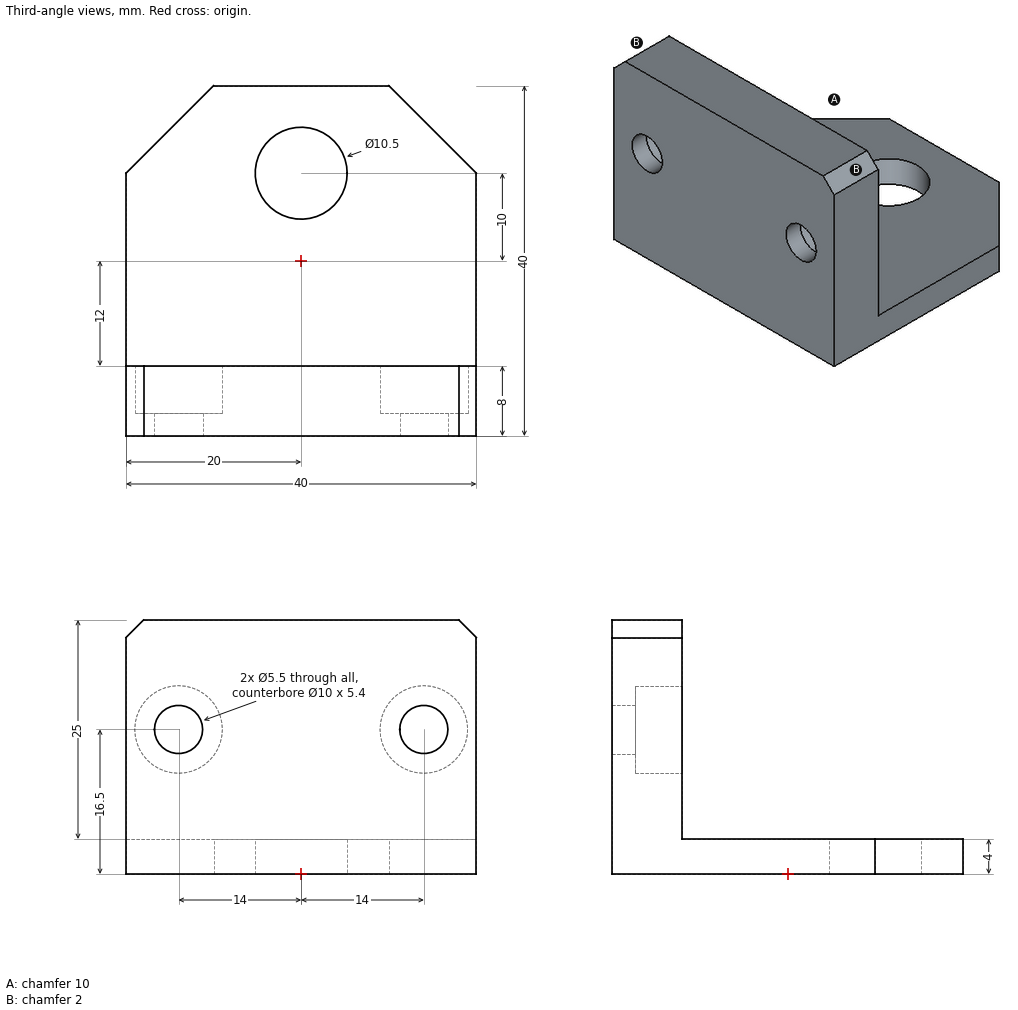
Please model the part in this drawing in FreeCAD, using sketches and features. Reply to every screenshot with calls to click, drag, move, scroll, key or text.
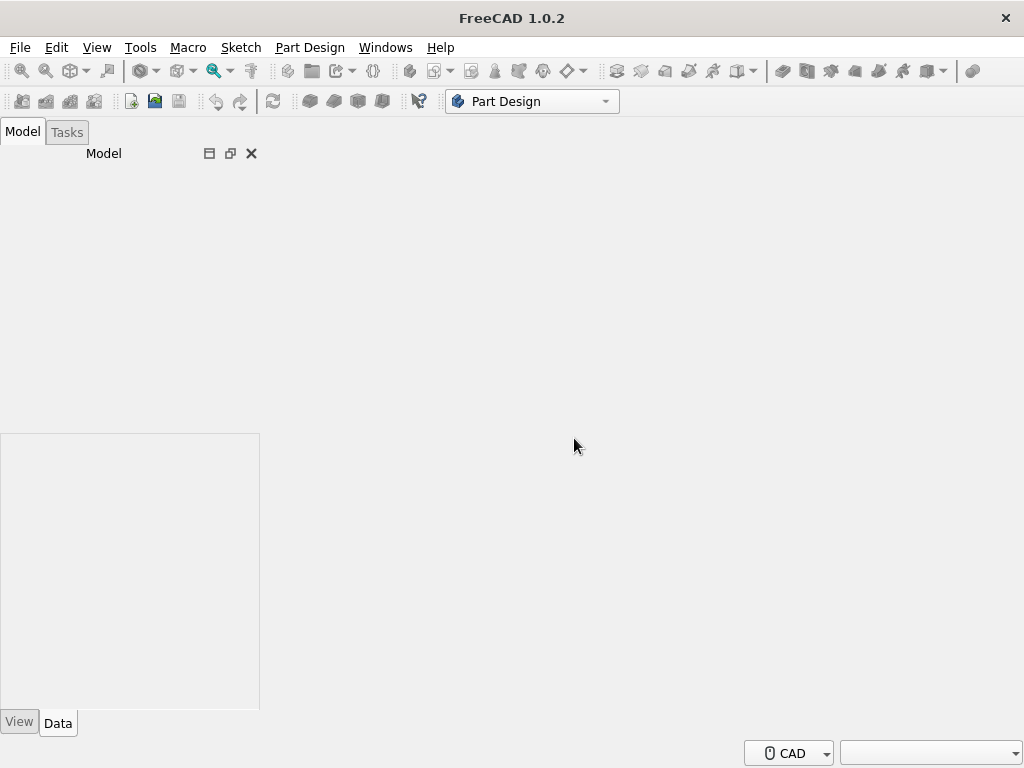
click(132, 102)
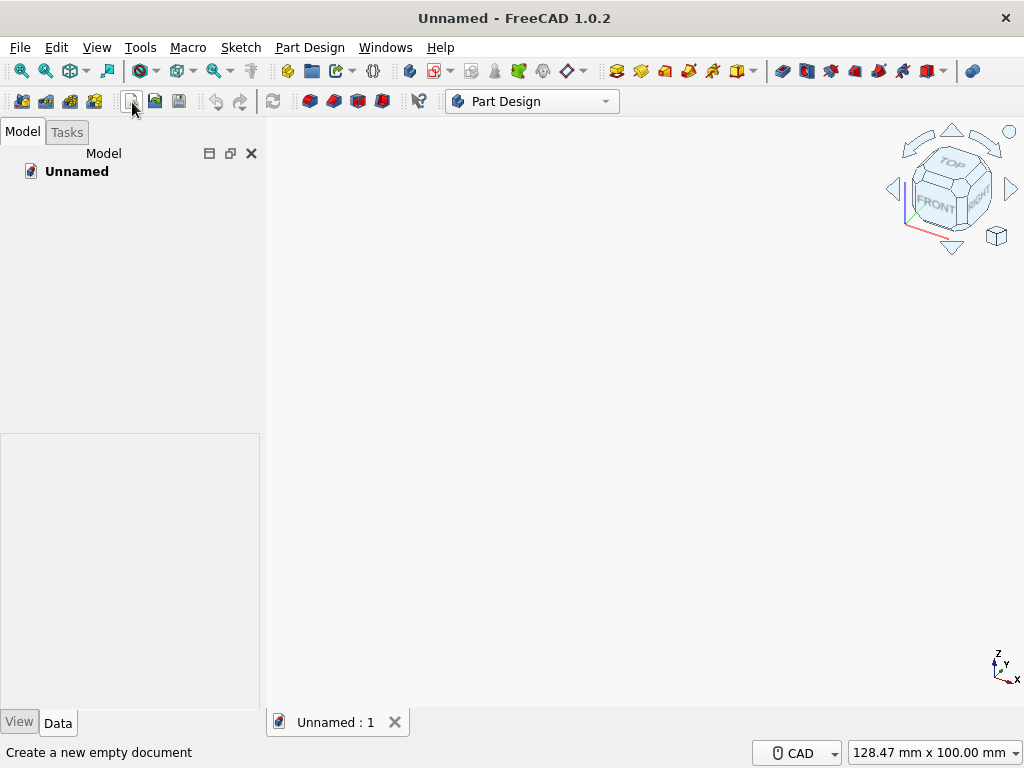
click(434, 72)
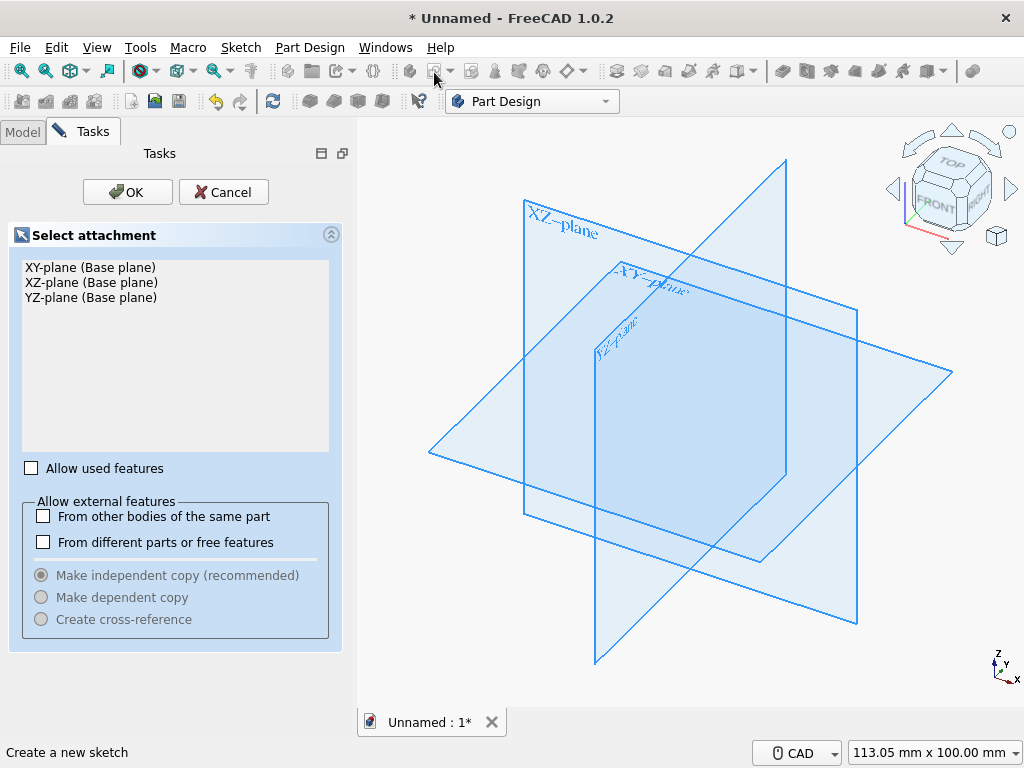
click(82, 268)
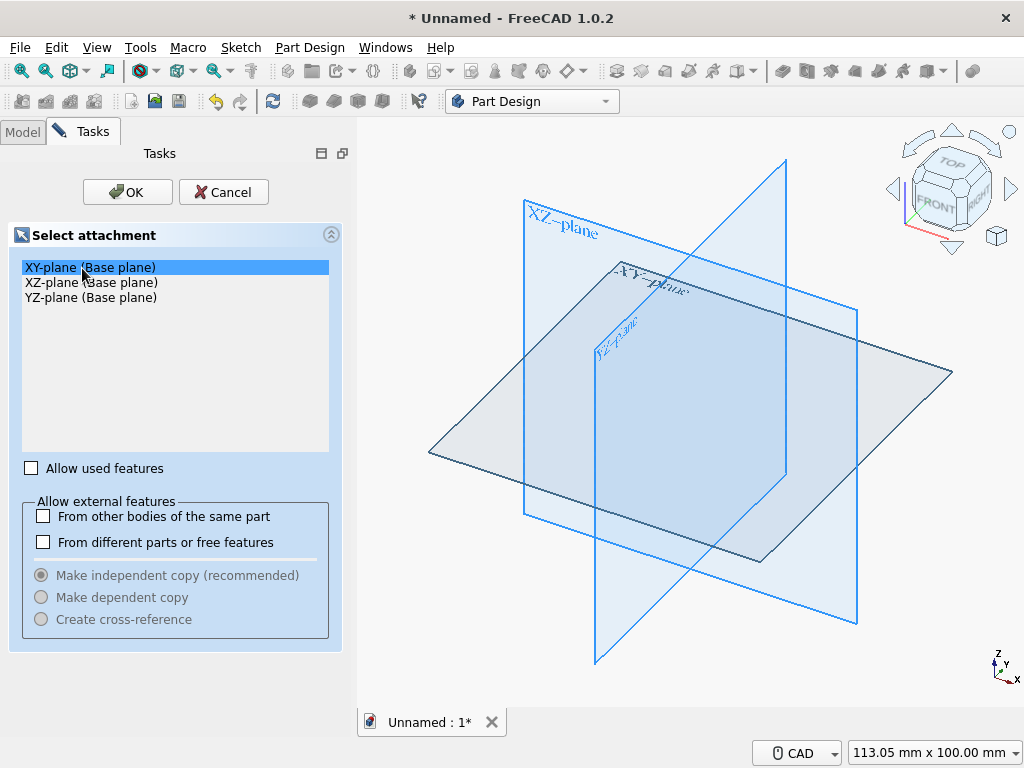
click(128, 192)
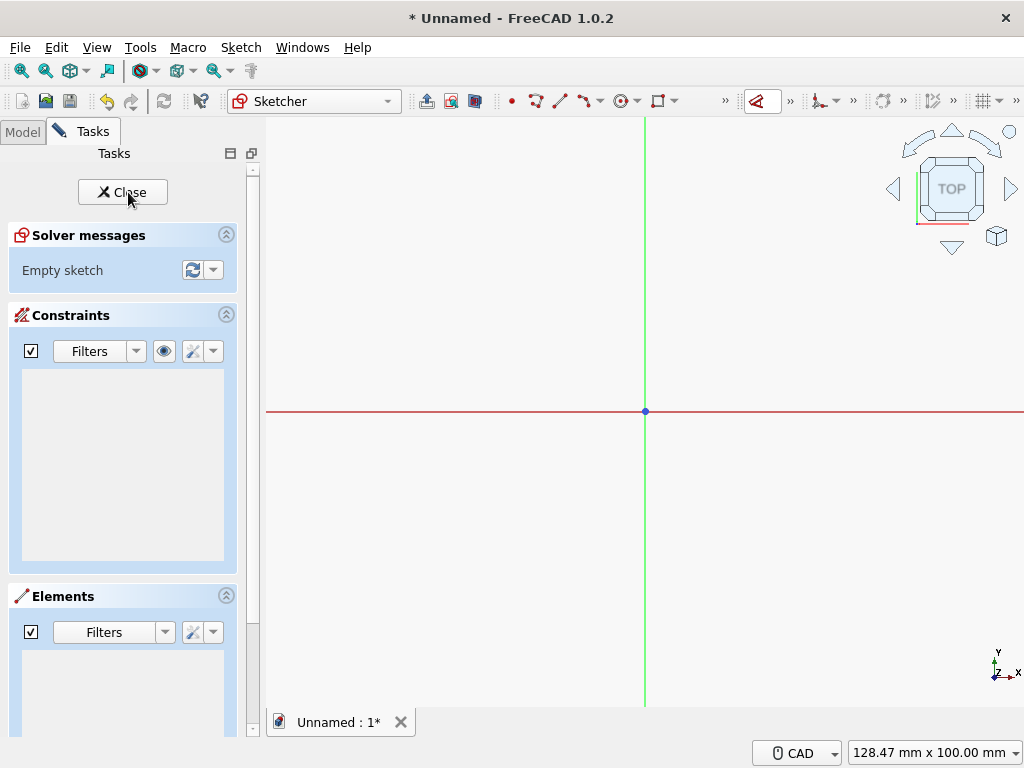
scroll(784, 412, up, 2)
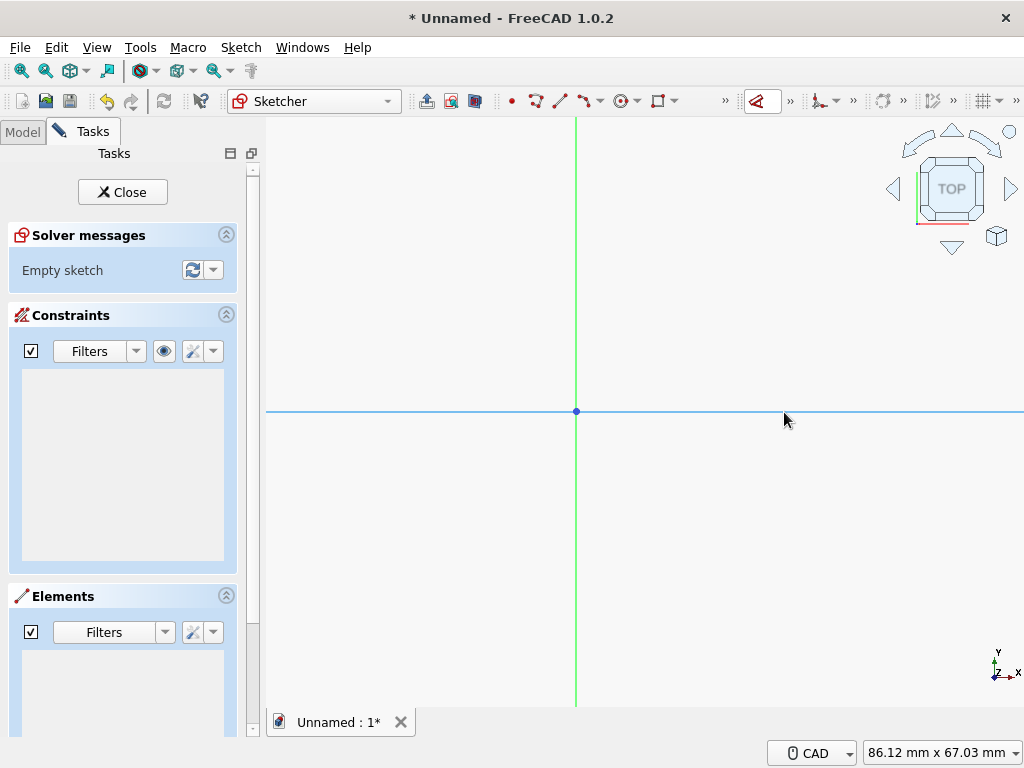
key(g)
key(v)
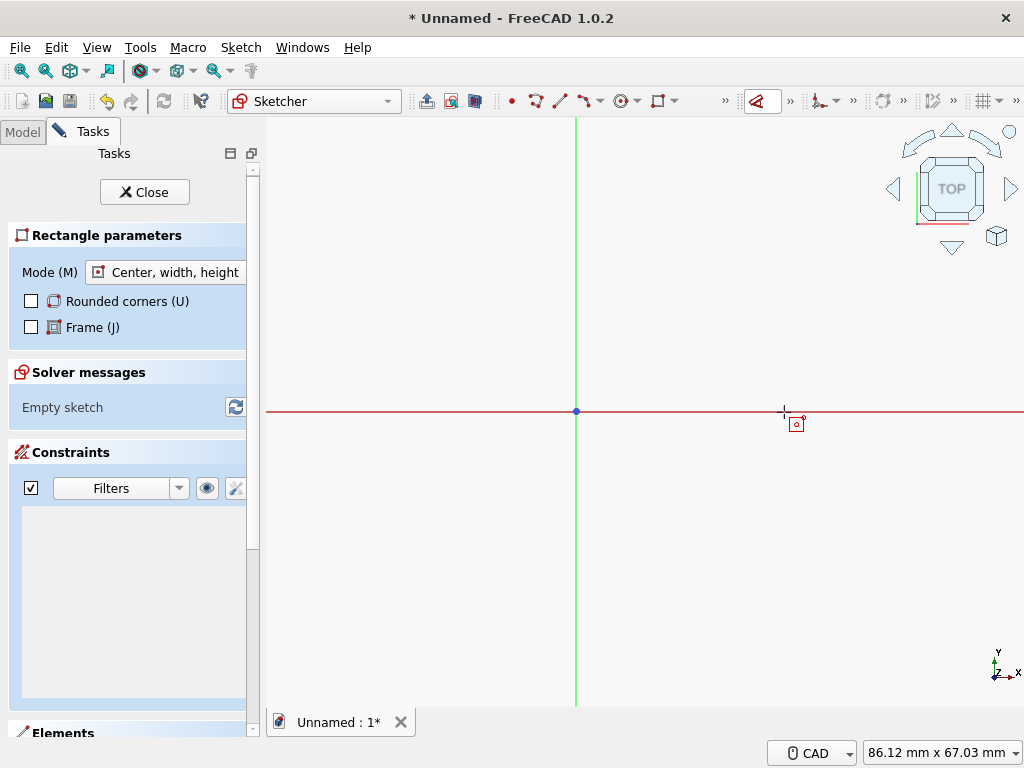
click(576, 412)
move(752, 236)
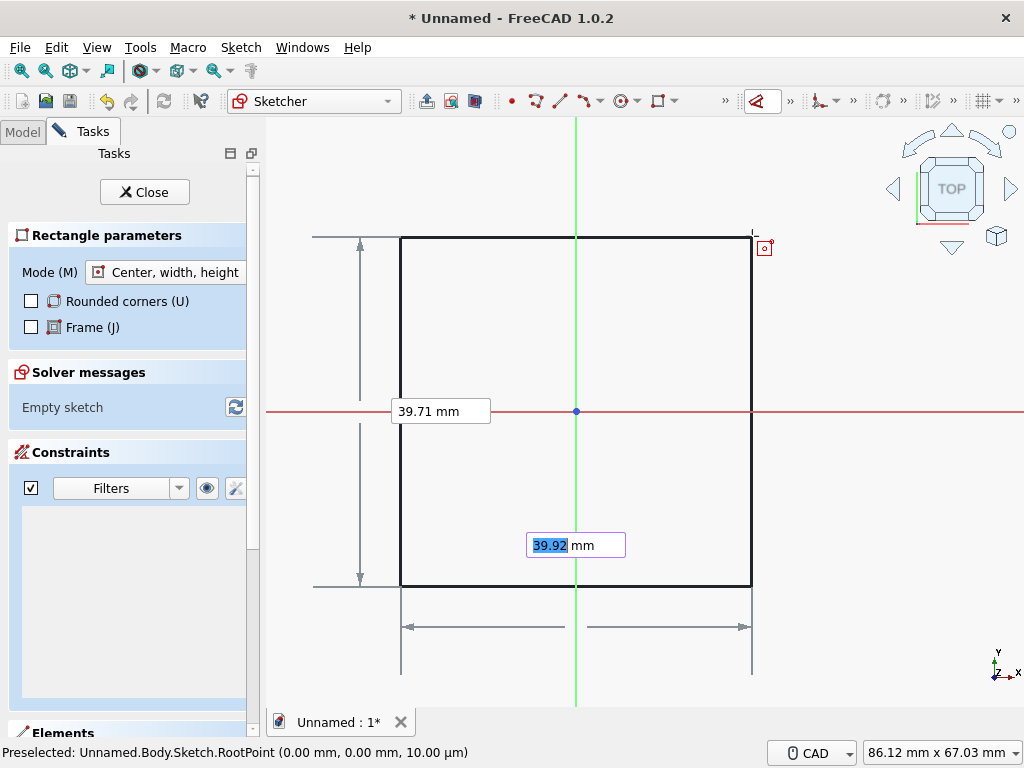
text(40)
key(Tab)
text(40)
key(Return)
key(Escape)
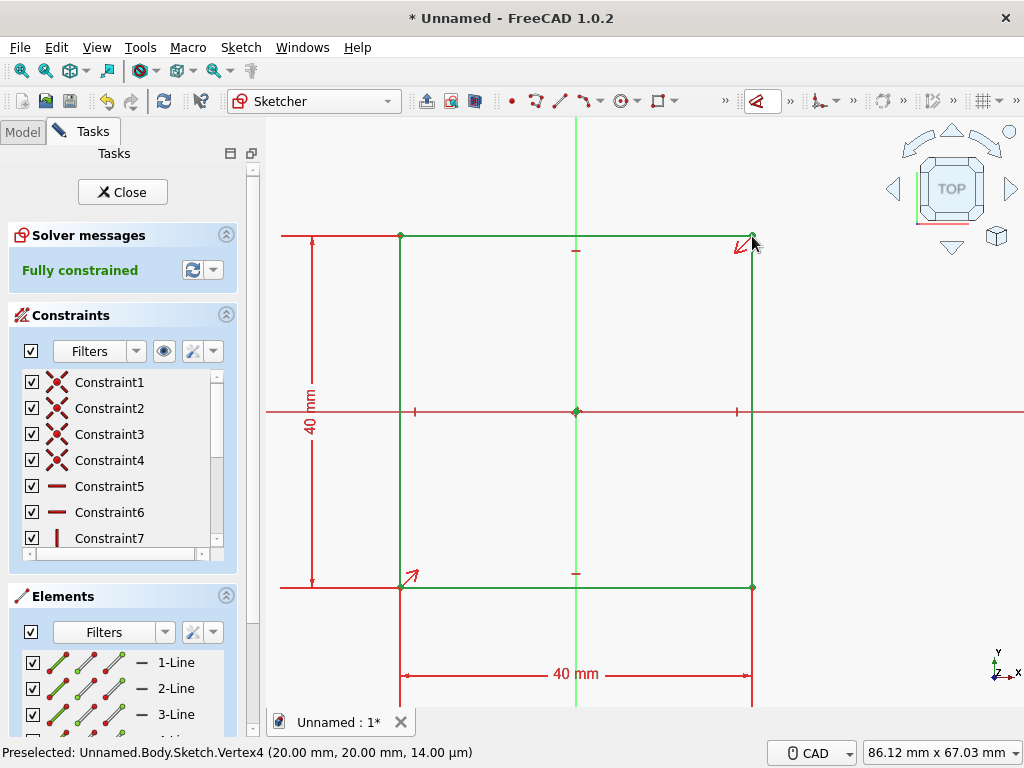
click(123, 192)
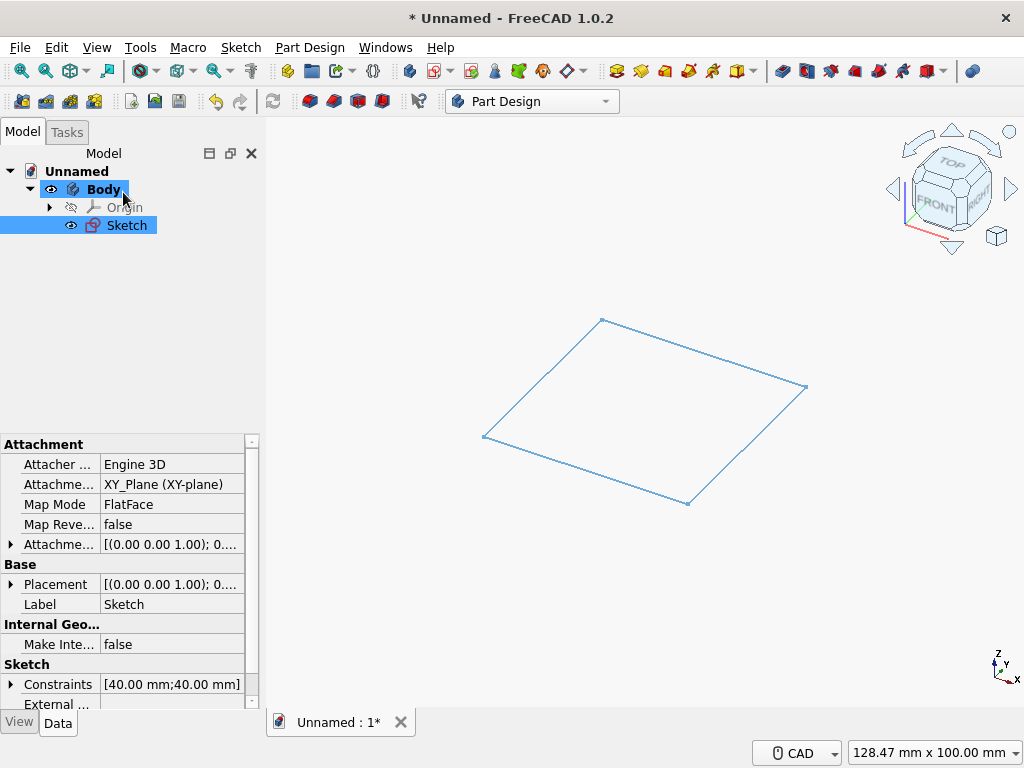
click(618, 72)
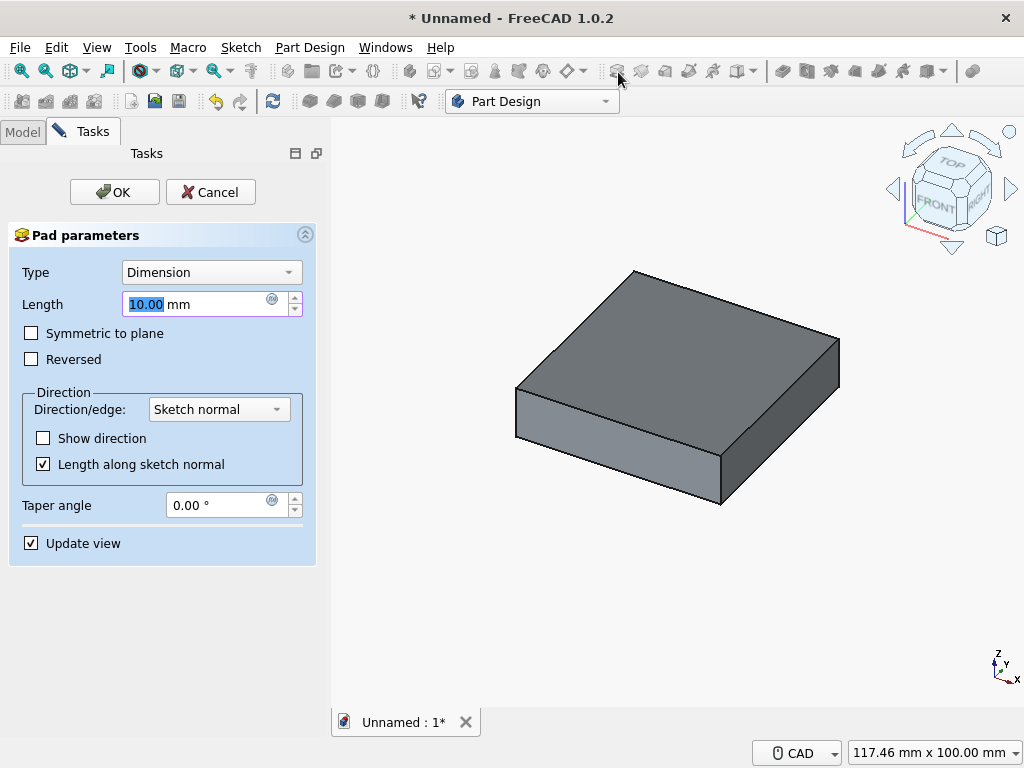
text(4)
key(Tab)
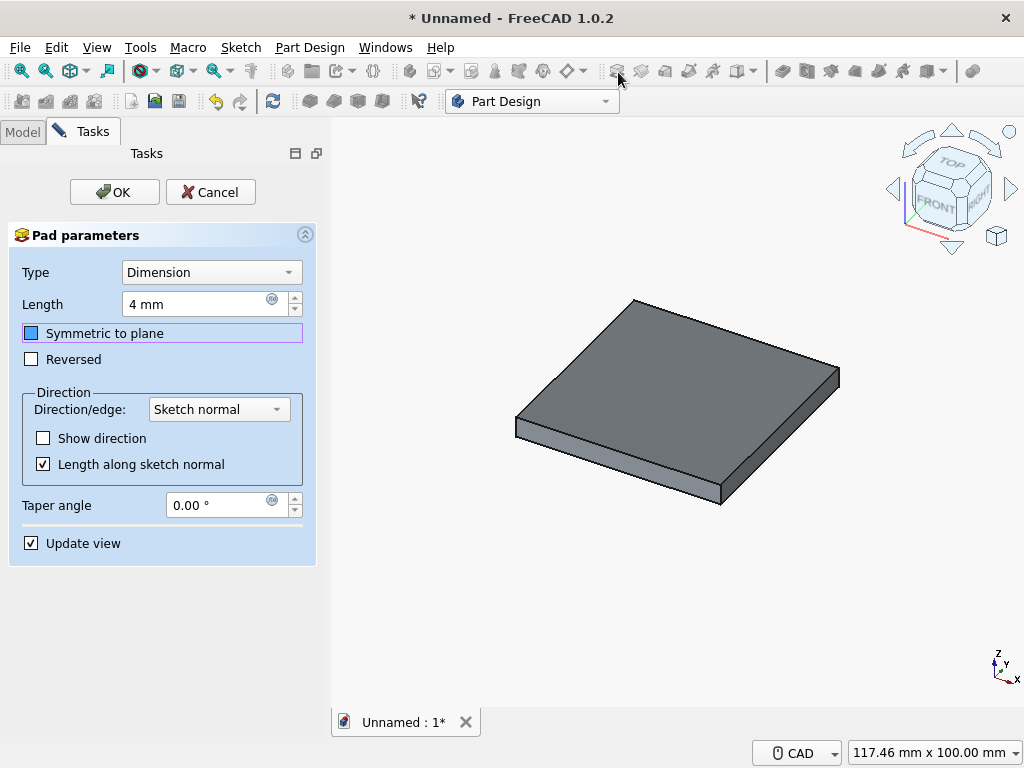
click(115, 192)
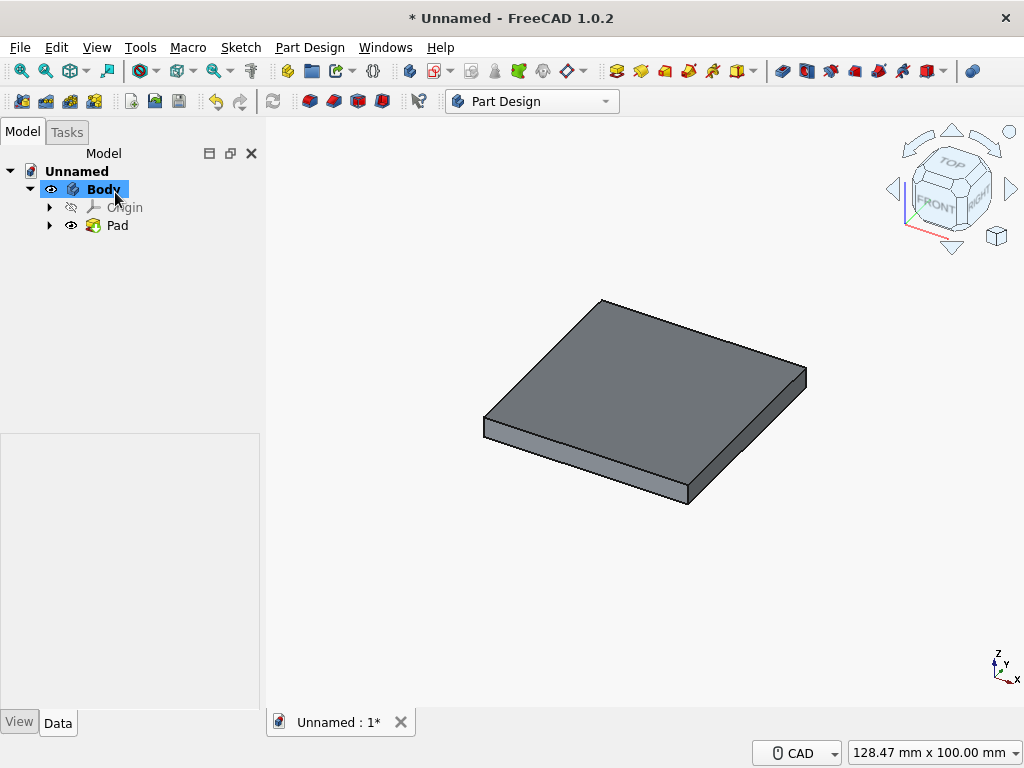
click(22, 72)